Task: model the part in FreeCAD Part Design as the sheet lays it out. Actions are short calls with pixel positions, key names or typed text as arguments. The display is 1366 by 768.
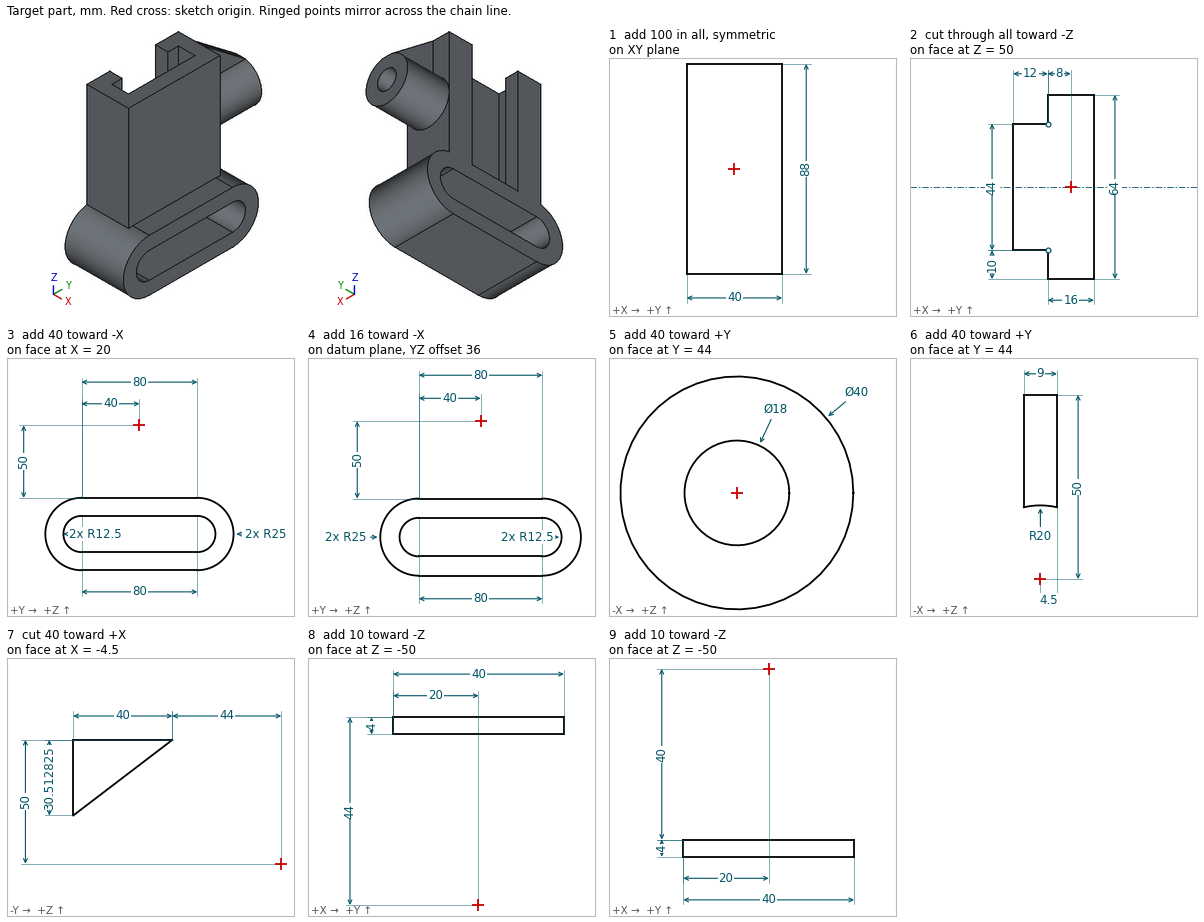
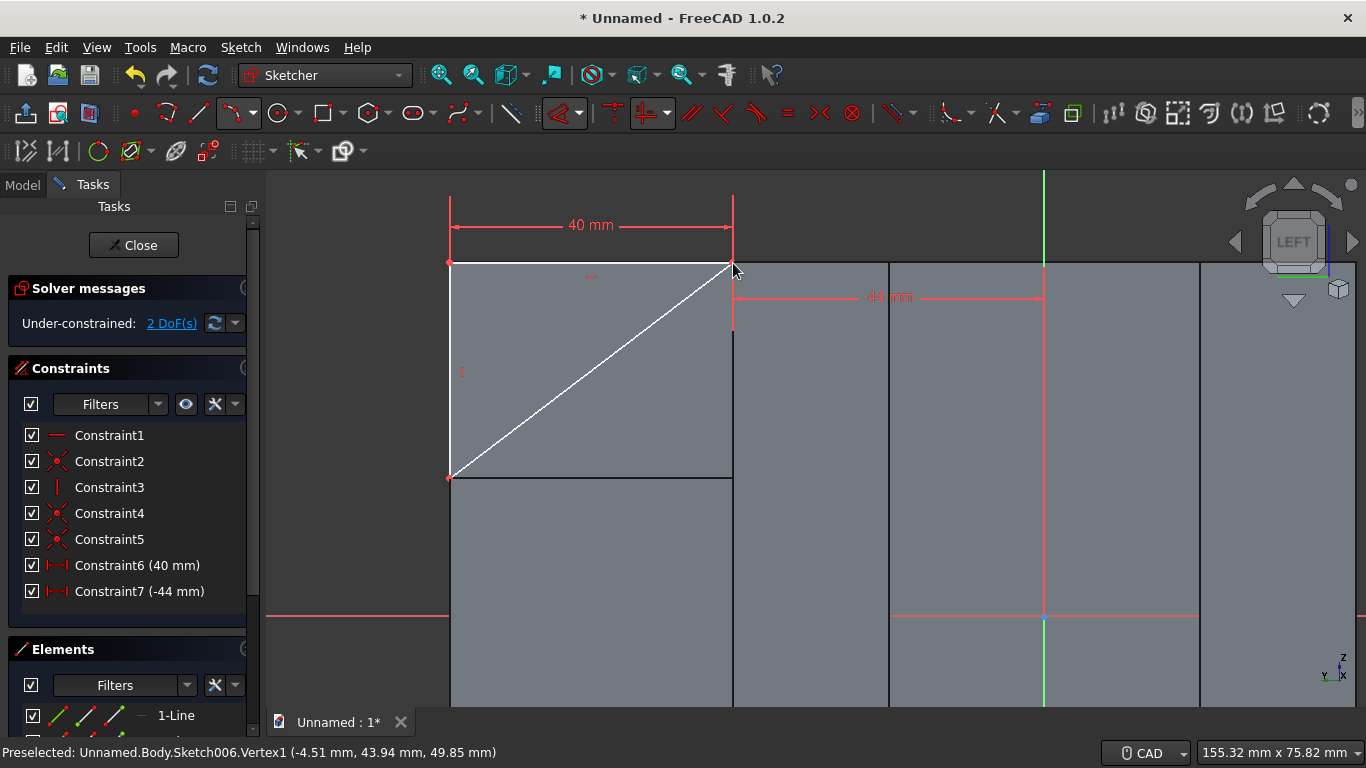
click(733, 263)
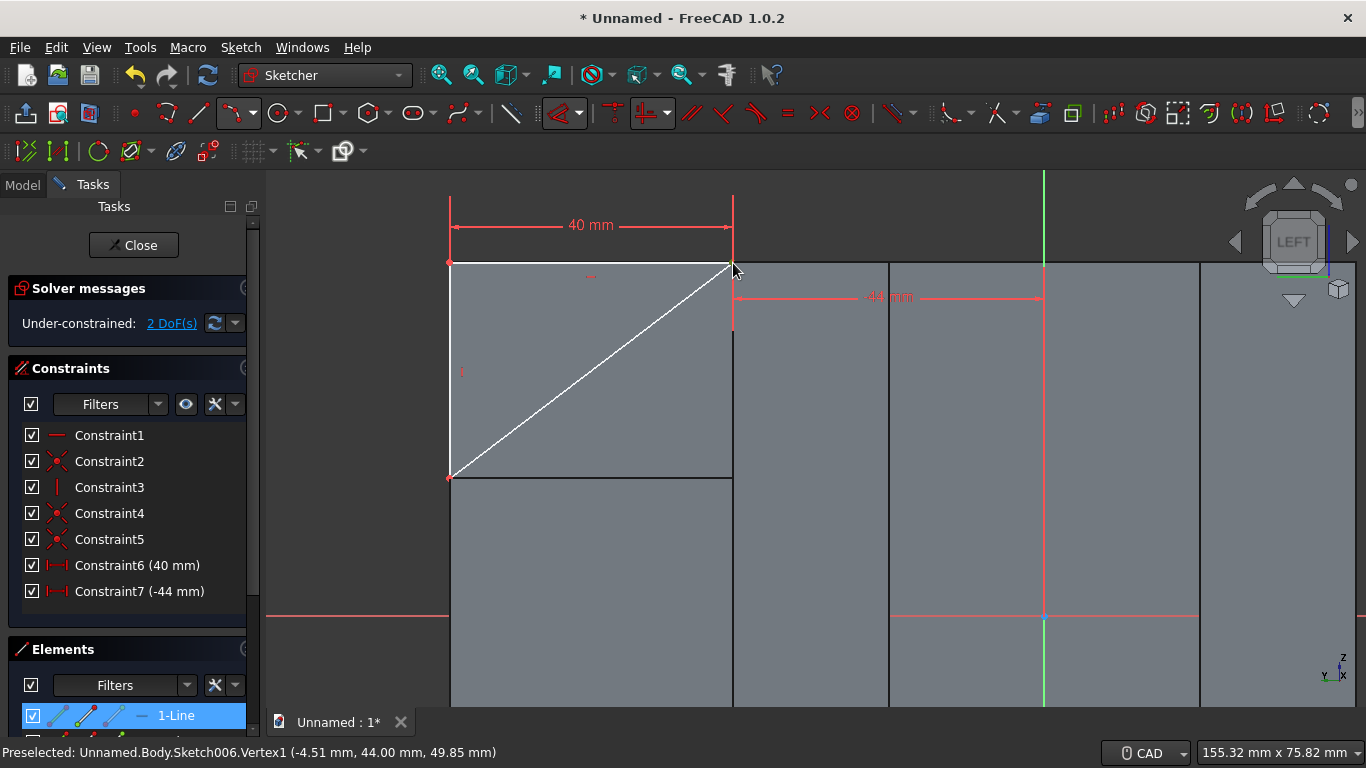
key(i)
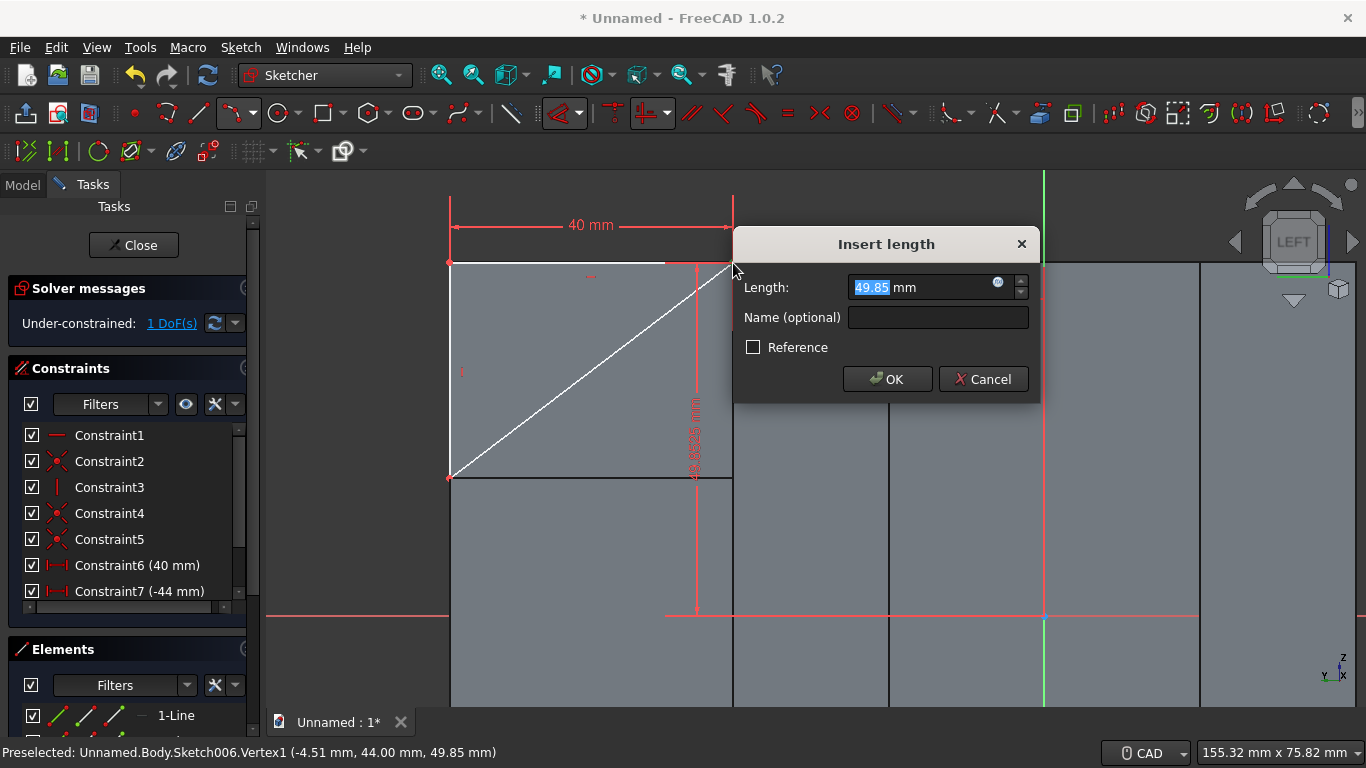
text(50)
key(Return)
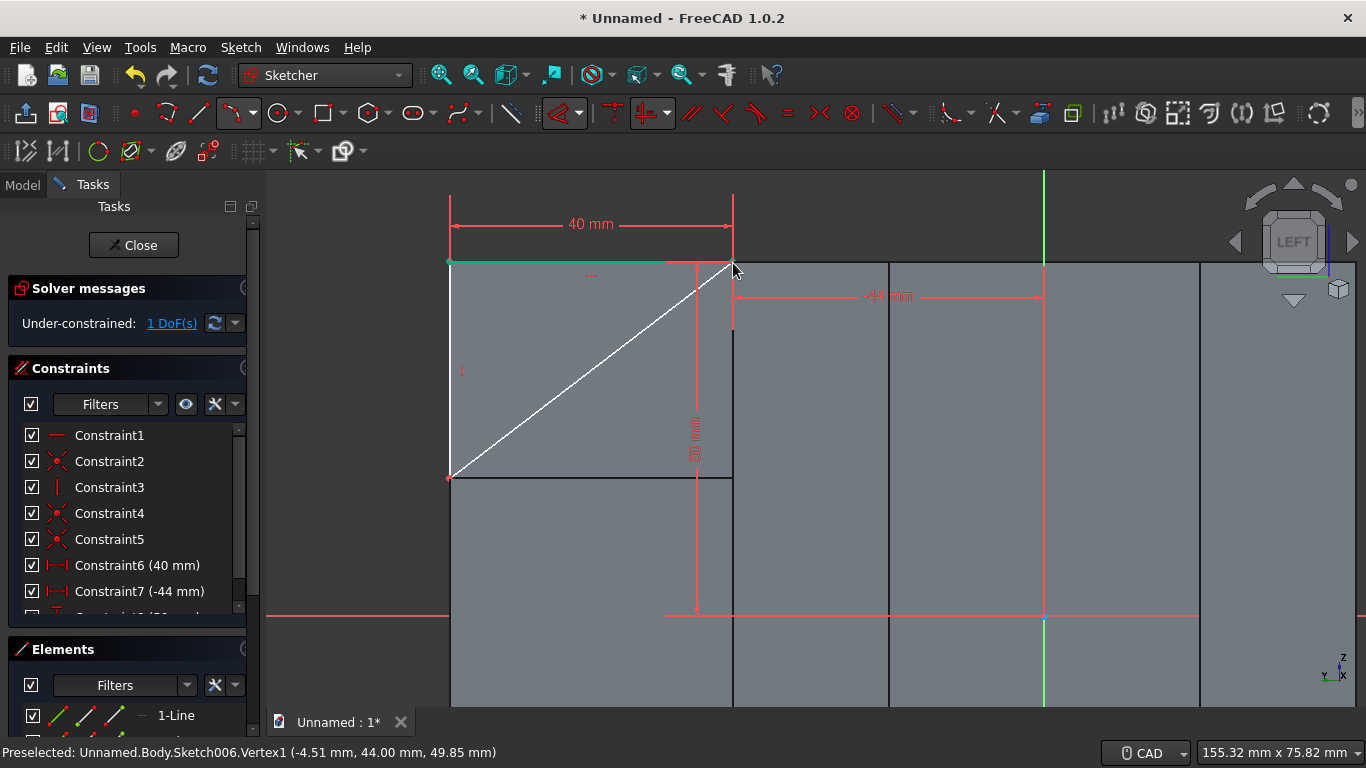
click(450, 327)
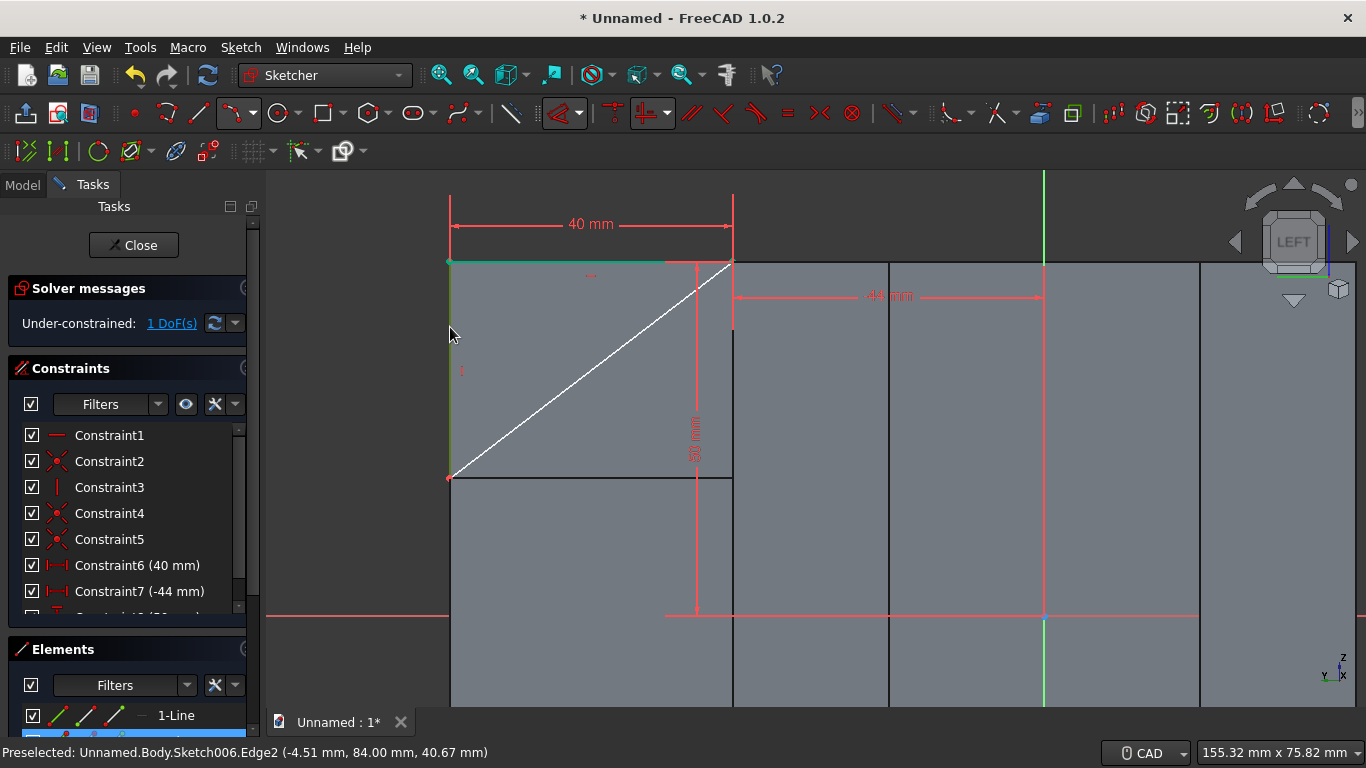
key(i)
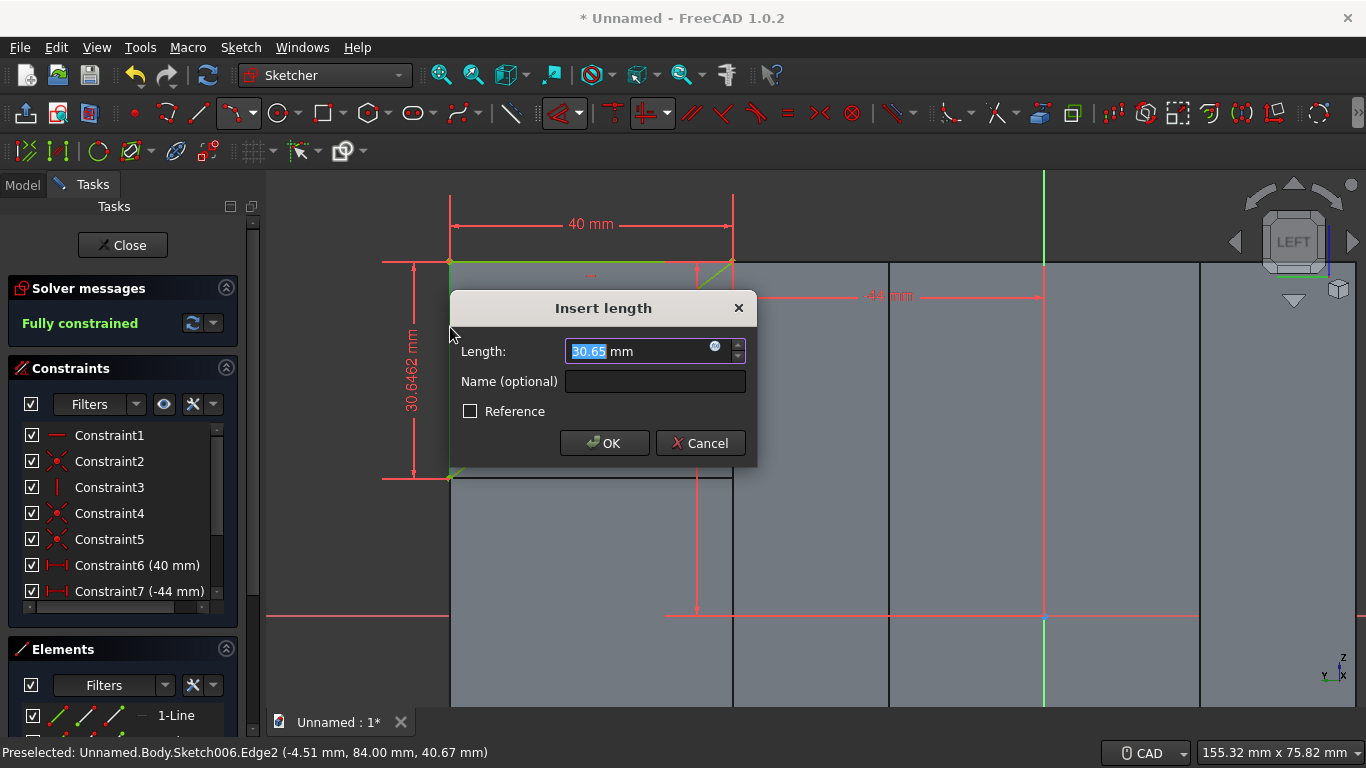
text(30.512825)
key(Return)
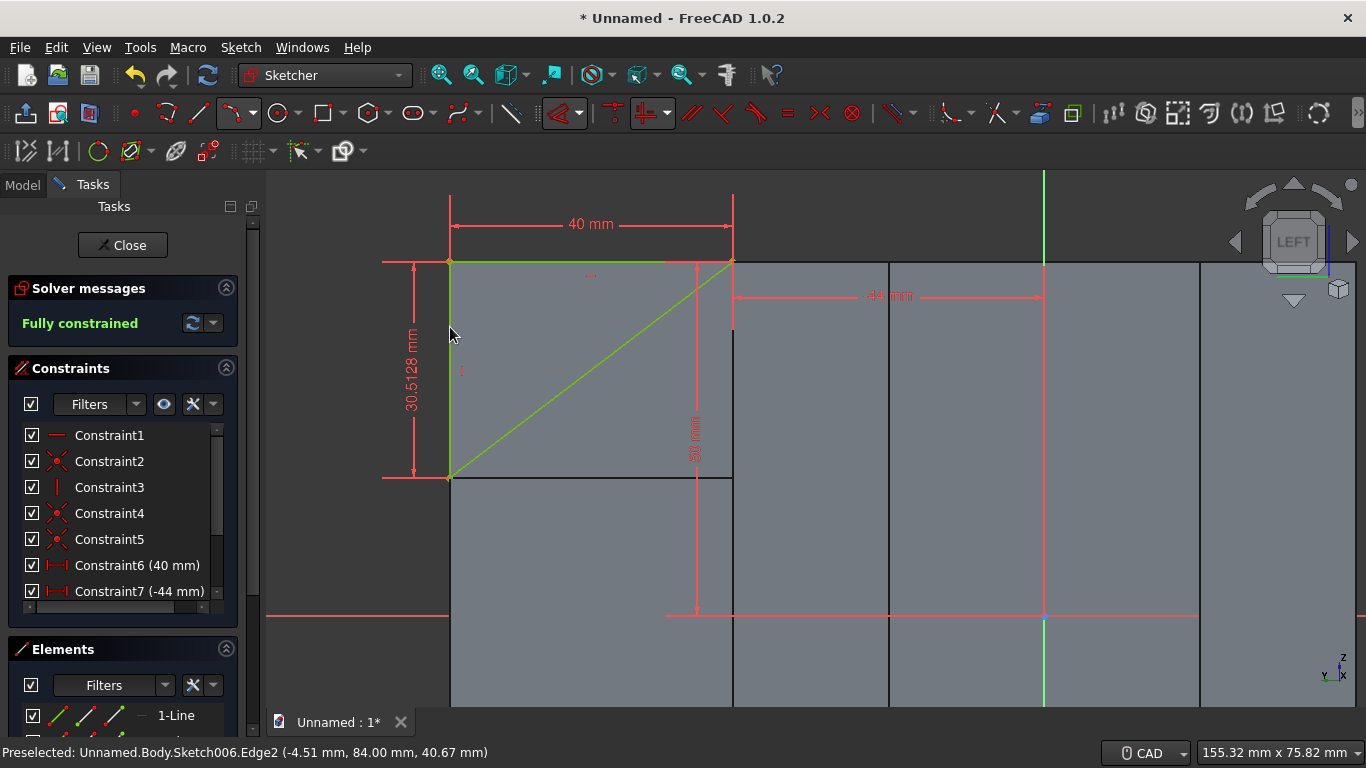
click(123, 245)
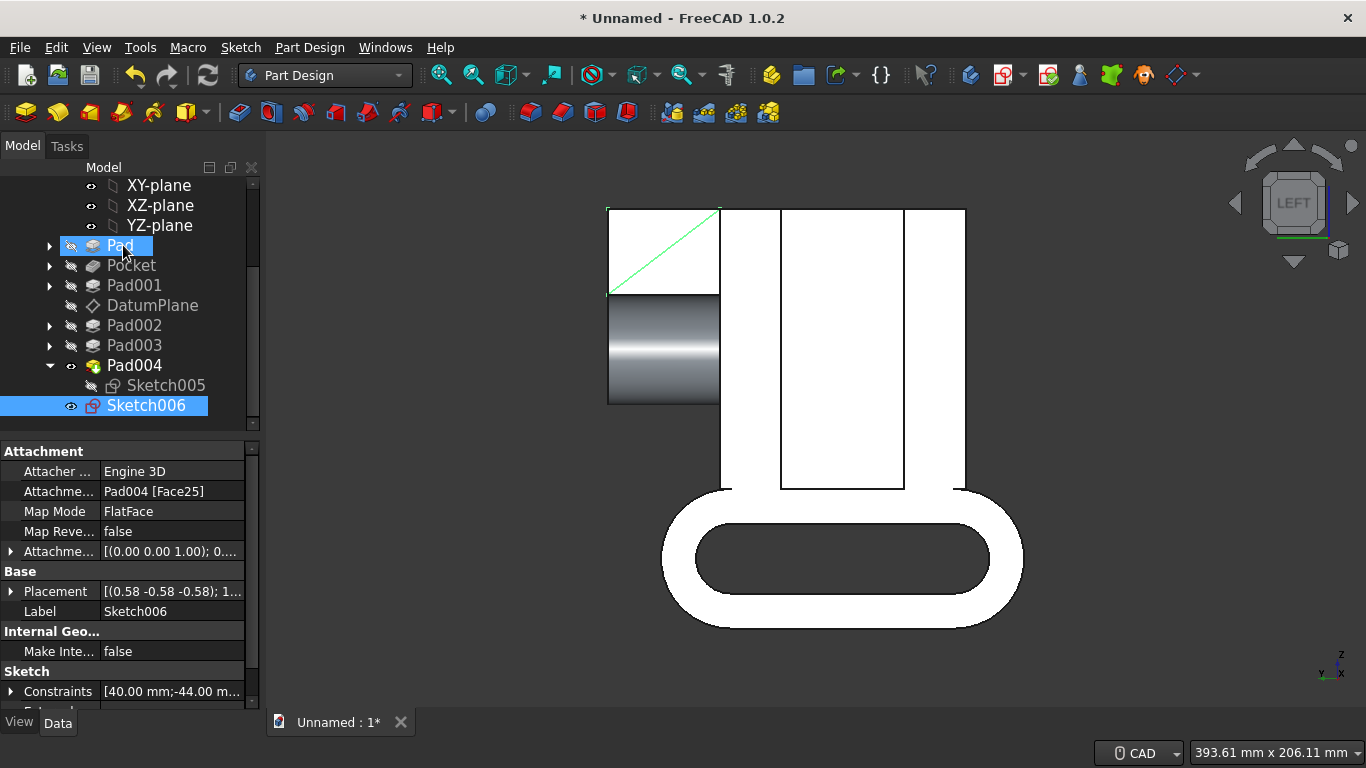
click(240, 112)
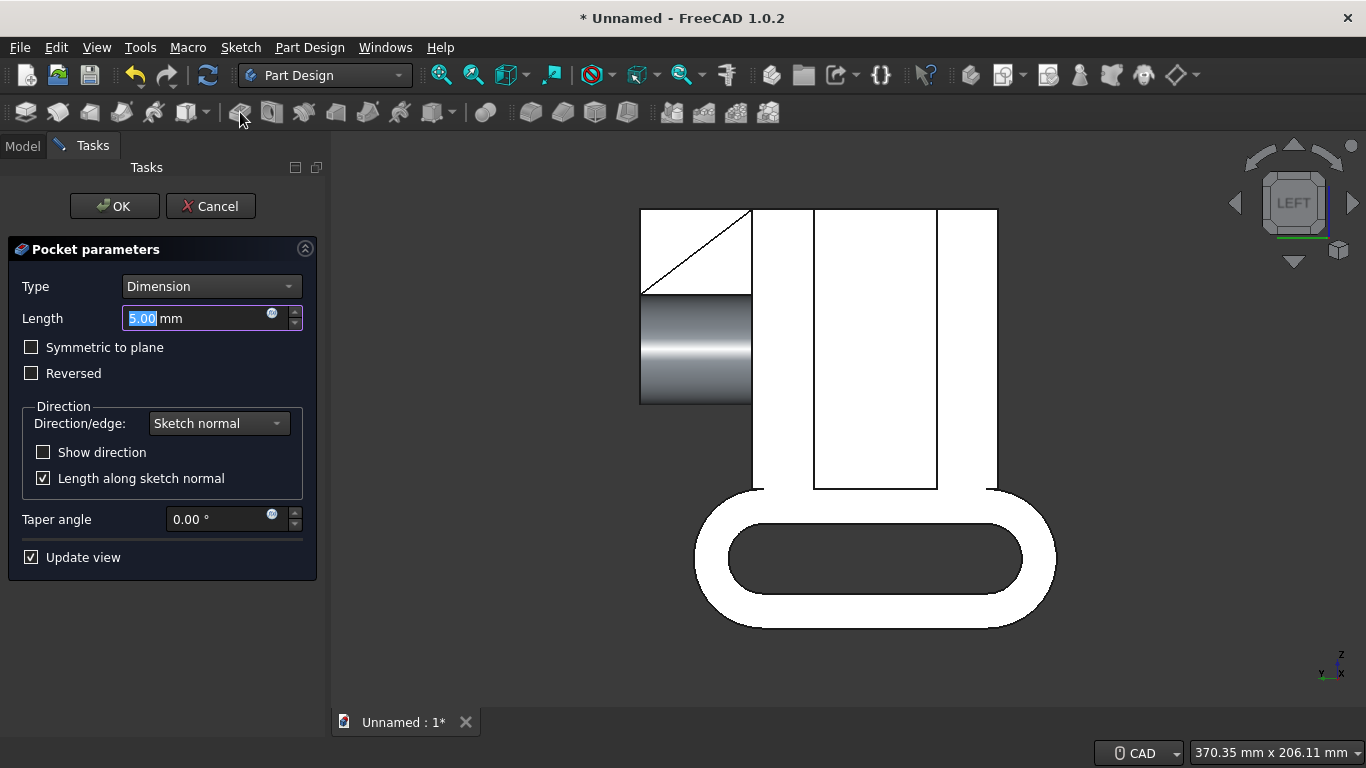
text(40)
key(Tab)